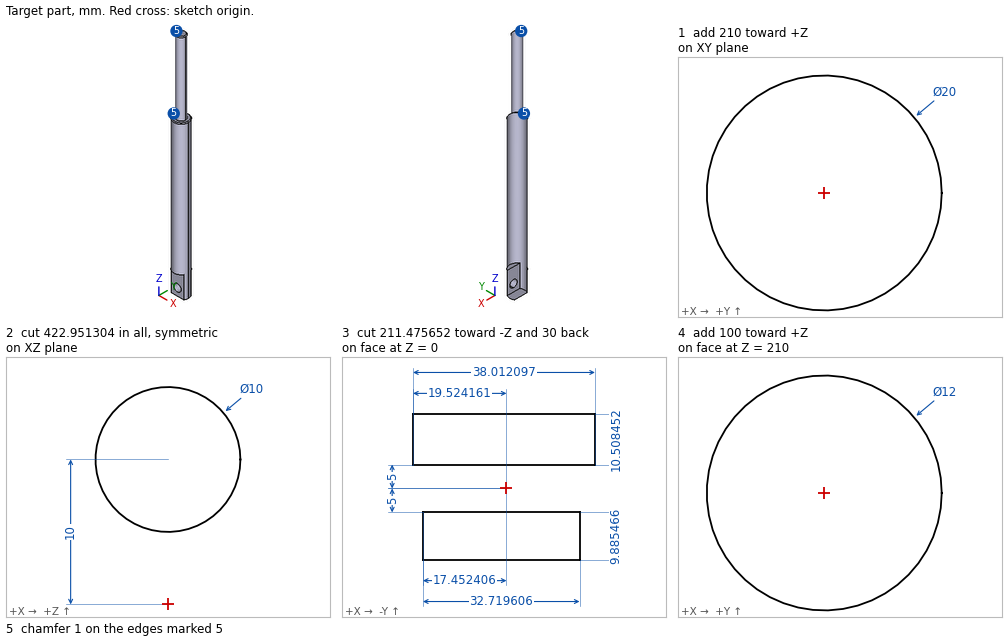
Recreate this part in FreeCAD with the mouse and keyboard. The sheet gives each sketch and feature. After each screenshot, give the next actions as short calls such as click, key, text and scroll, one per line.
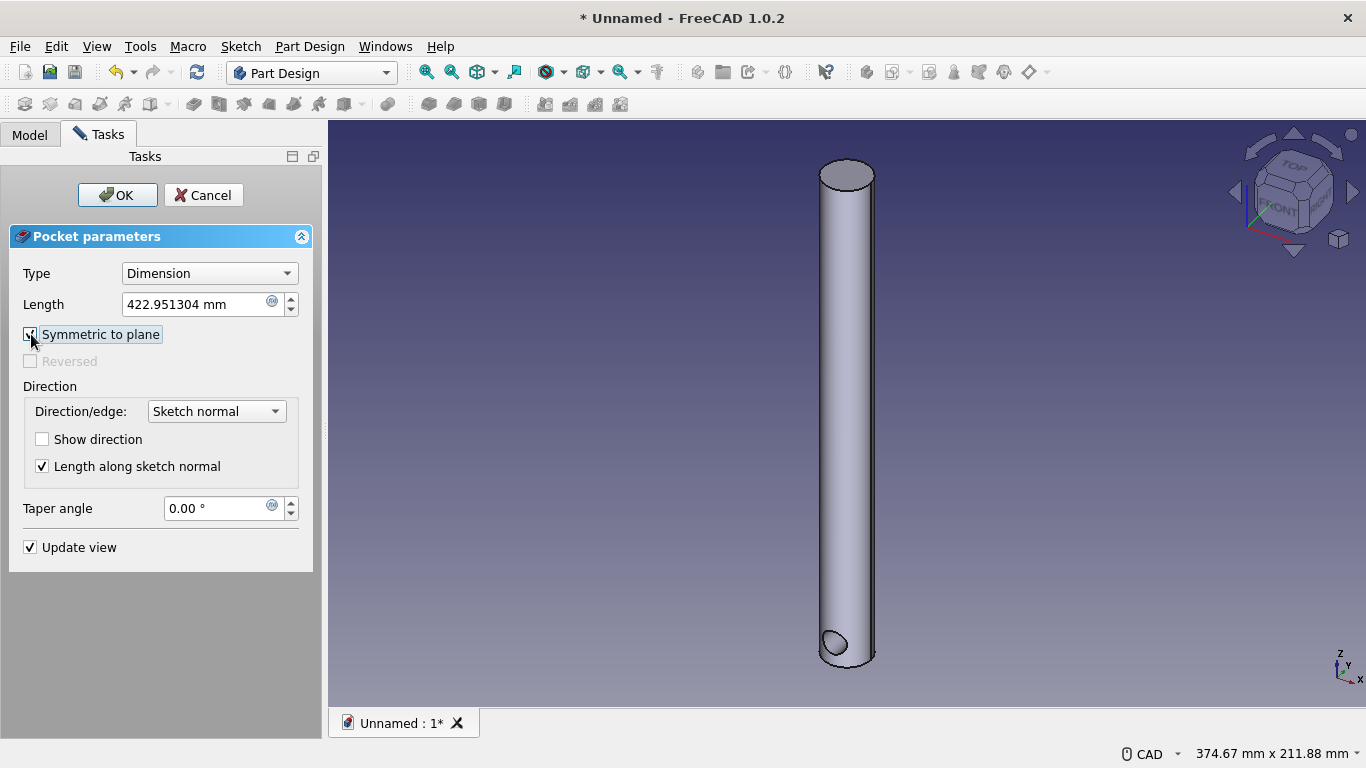
click(118, 195)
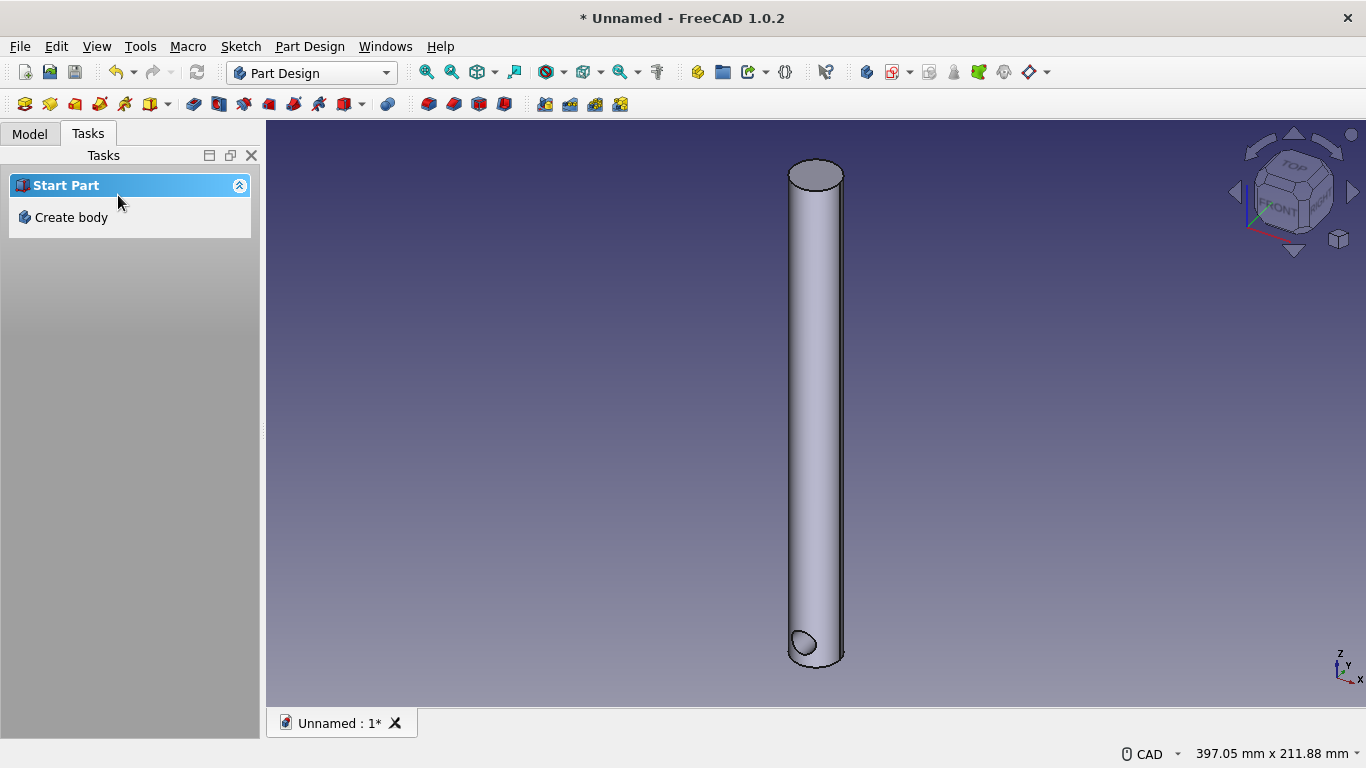
key(5)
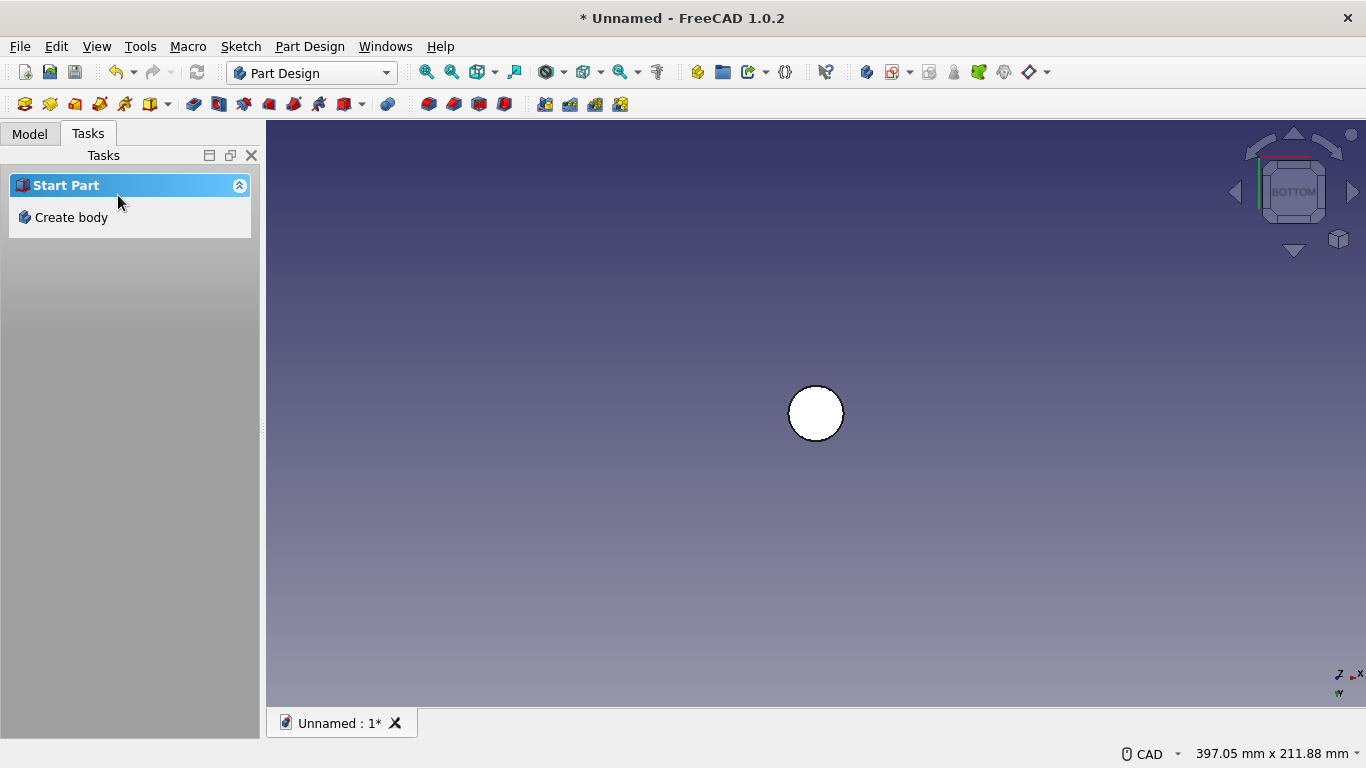
click(427, 72)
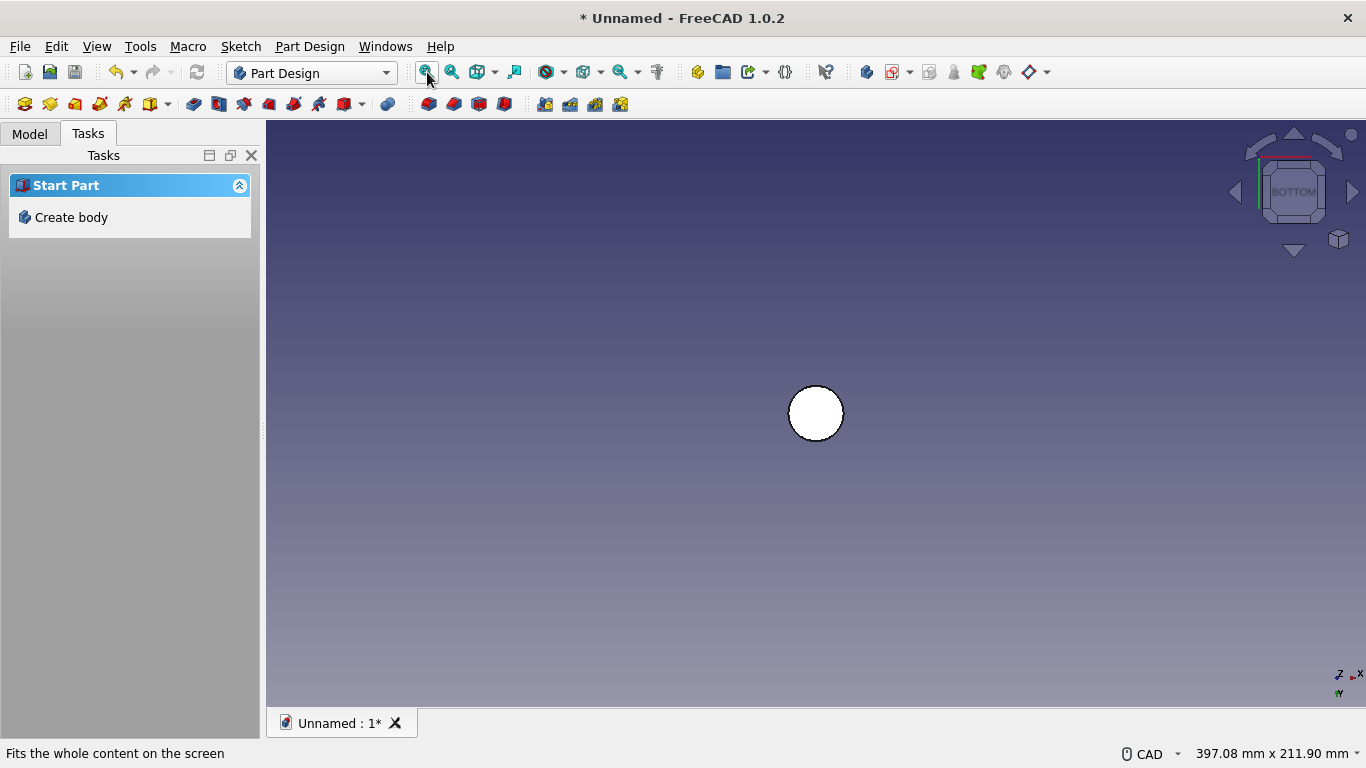
click(816, 412)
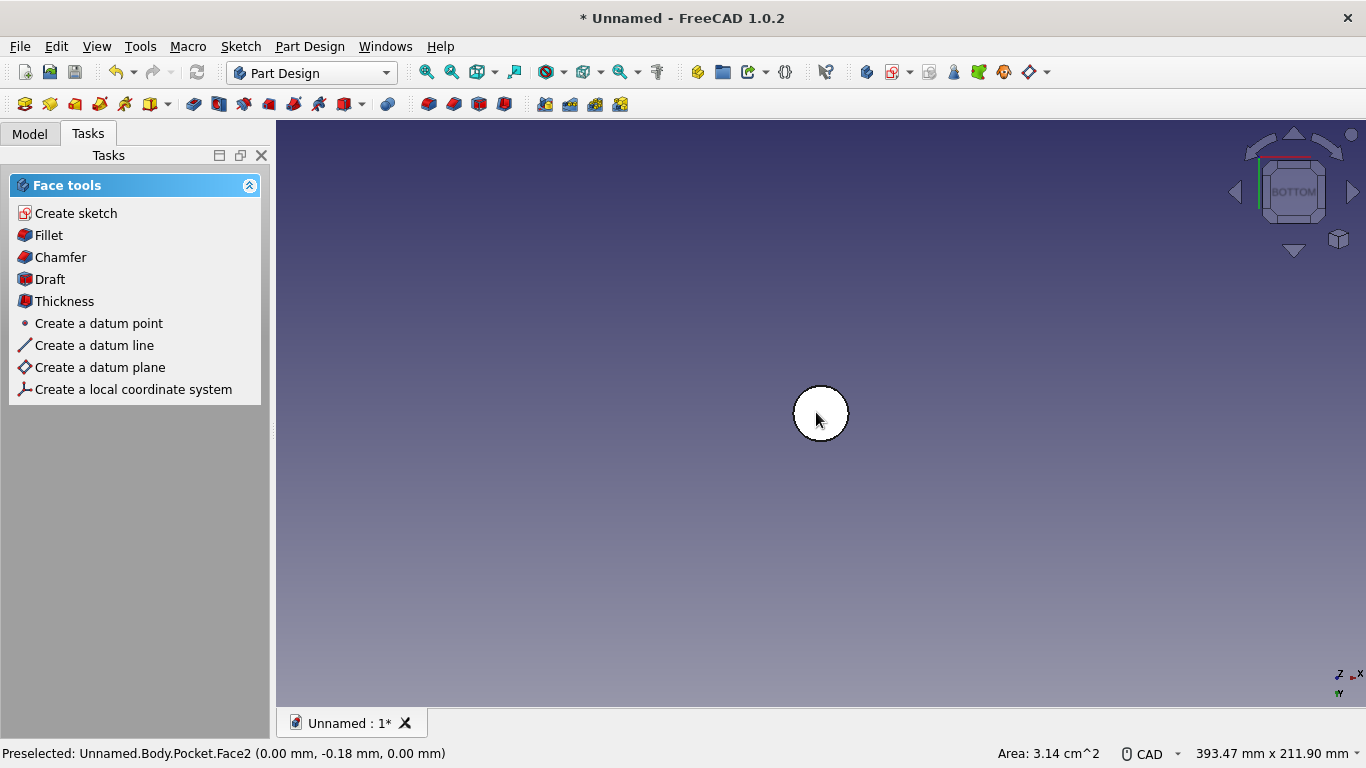
click(892, 72)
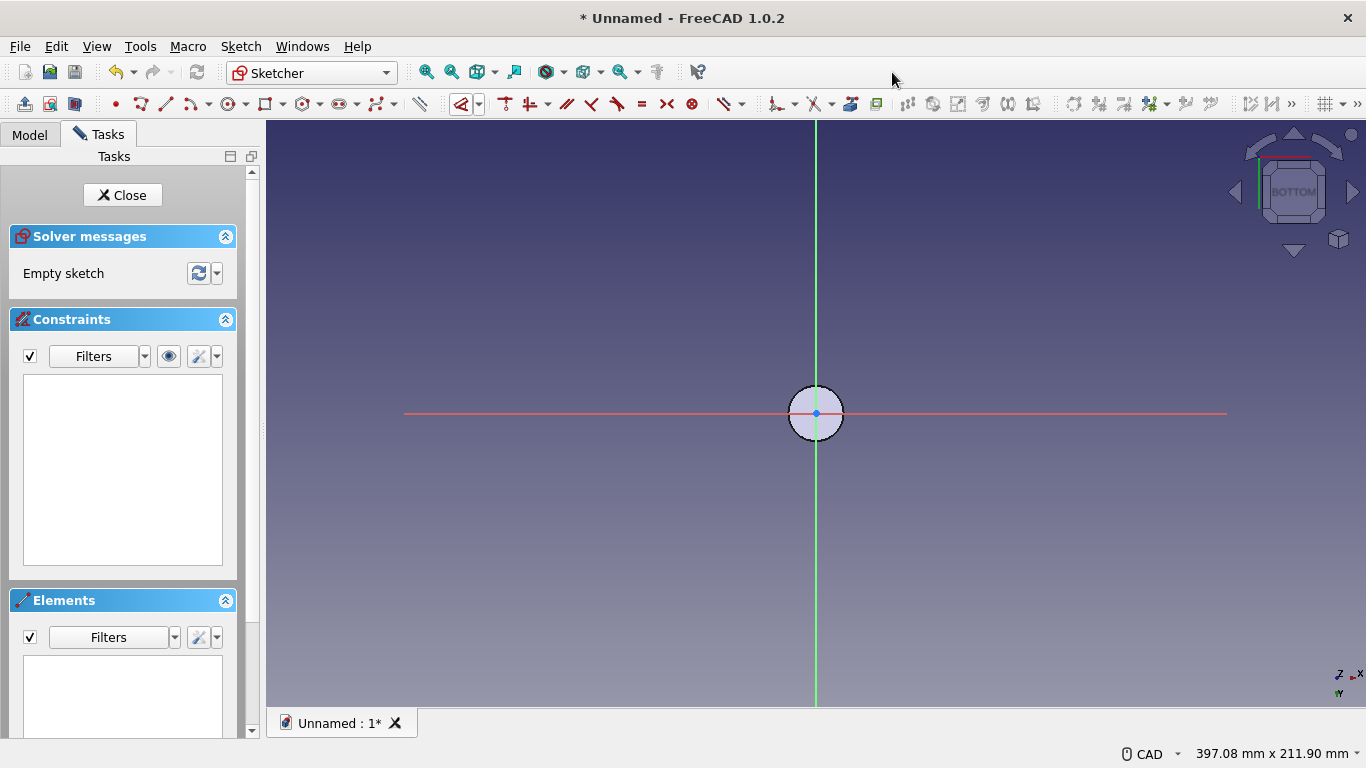
scroll(837, 412, up, 7)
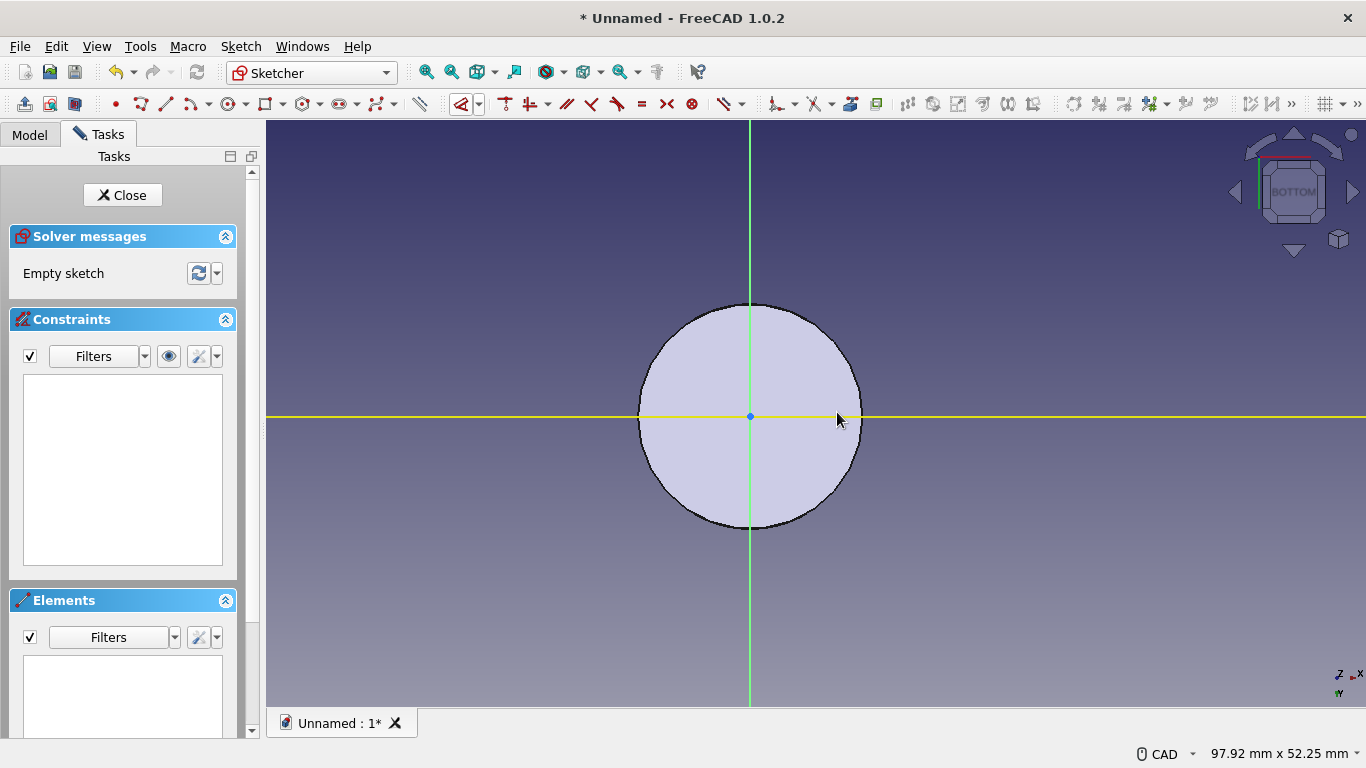
click(264, 104)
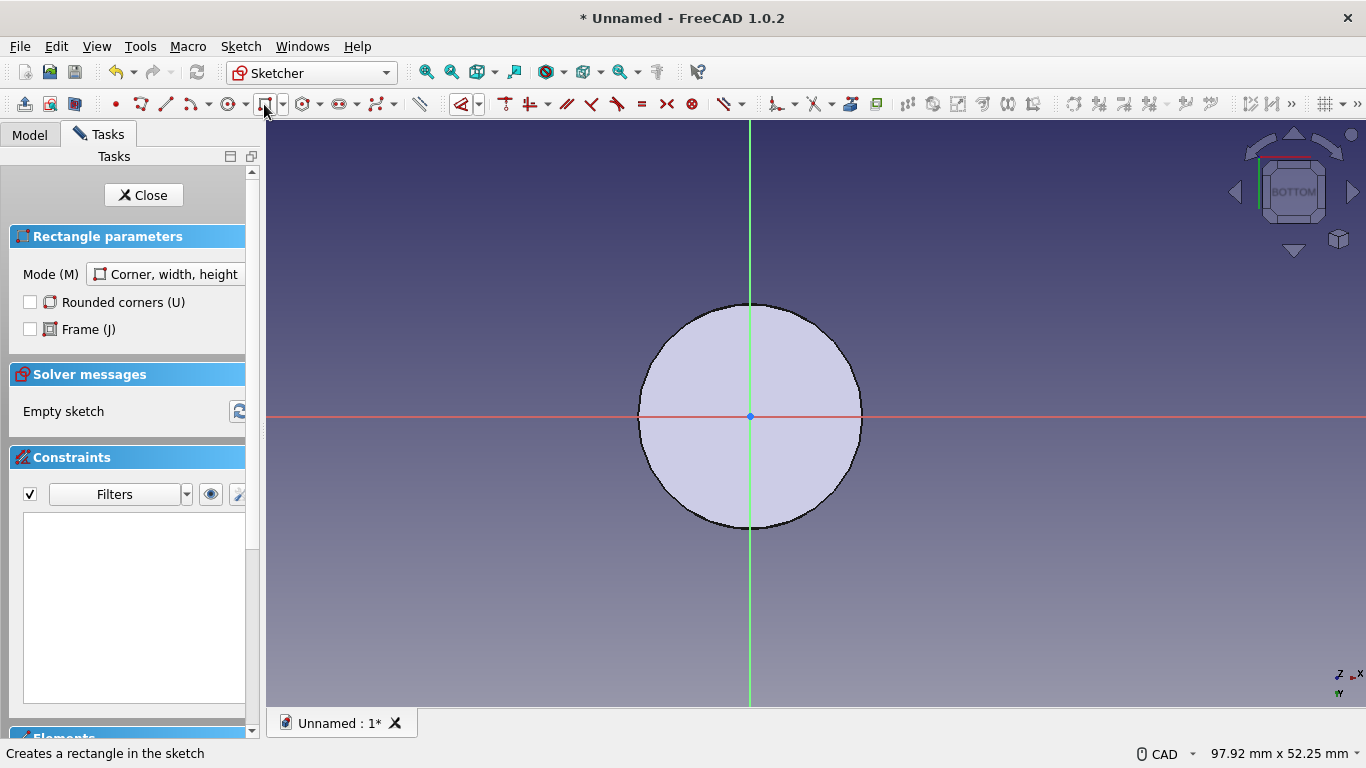
click(531, 242)
move(958, 360)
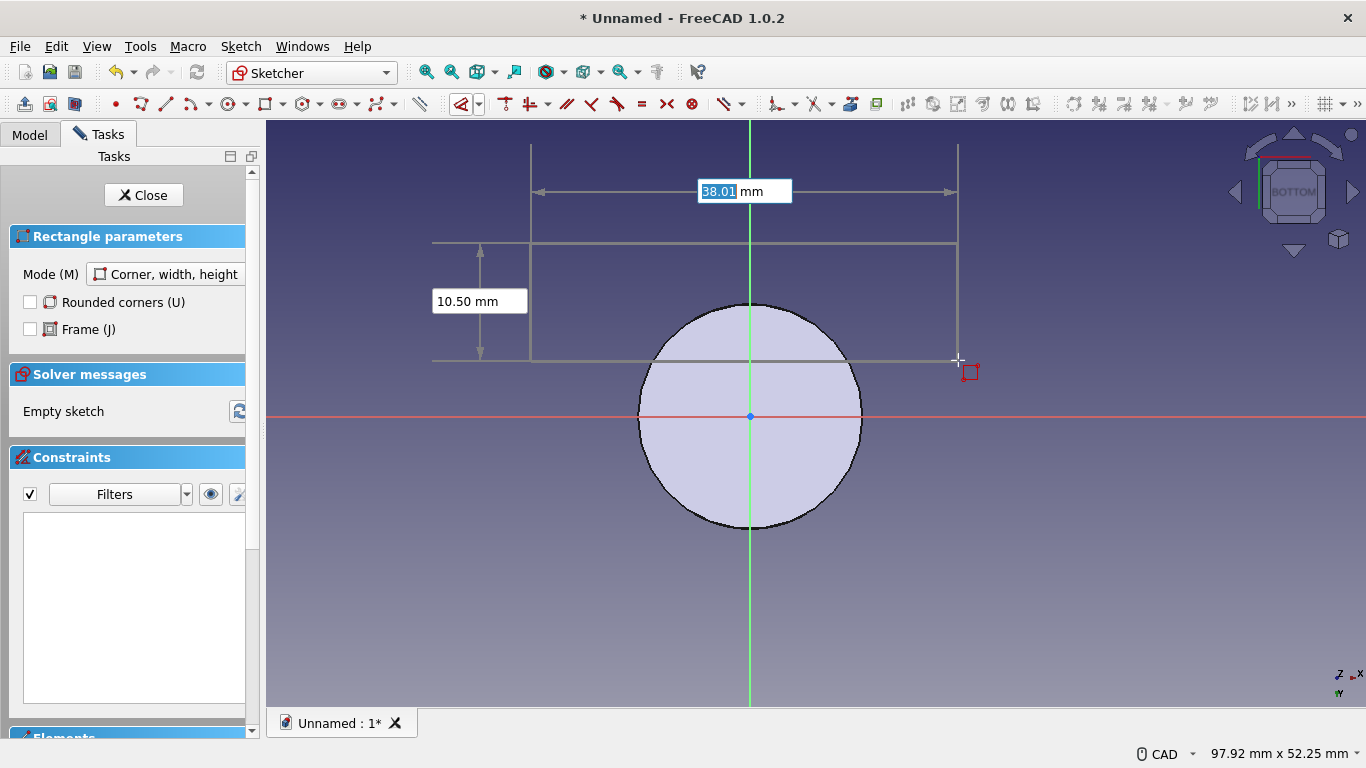
text(38.012097)
key(Tab)
text(10.508452)
key(Return)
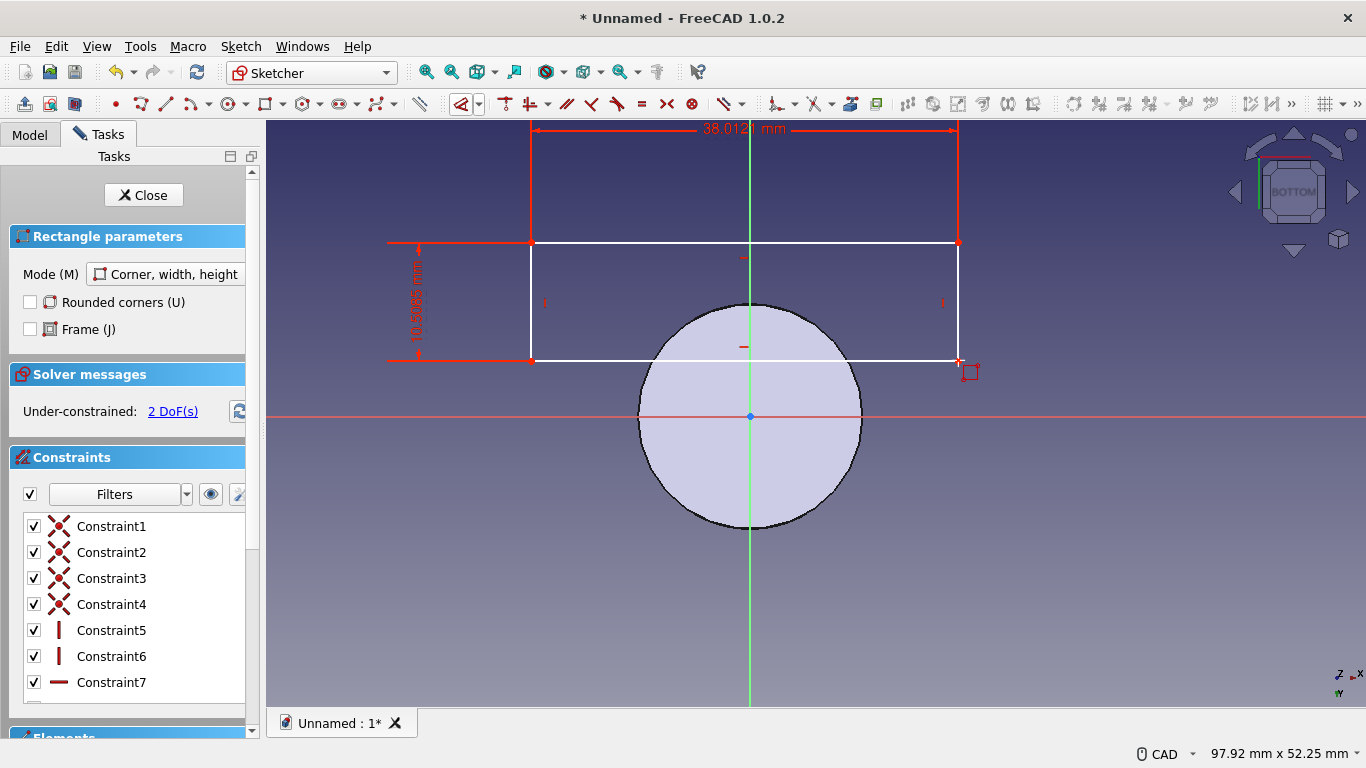
click(554, 473)
move(922, 584)